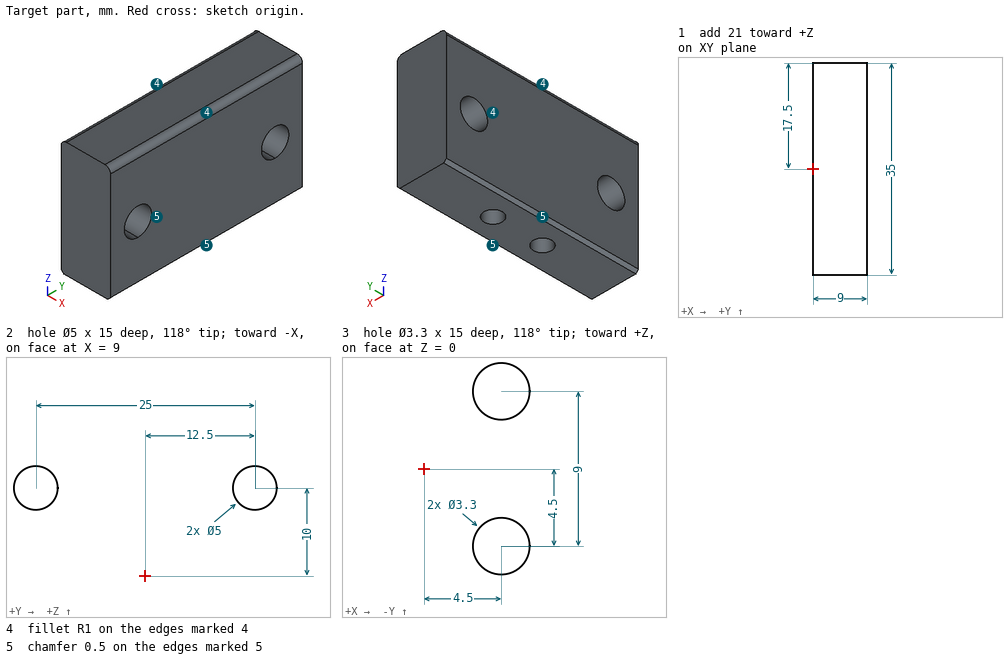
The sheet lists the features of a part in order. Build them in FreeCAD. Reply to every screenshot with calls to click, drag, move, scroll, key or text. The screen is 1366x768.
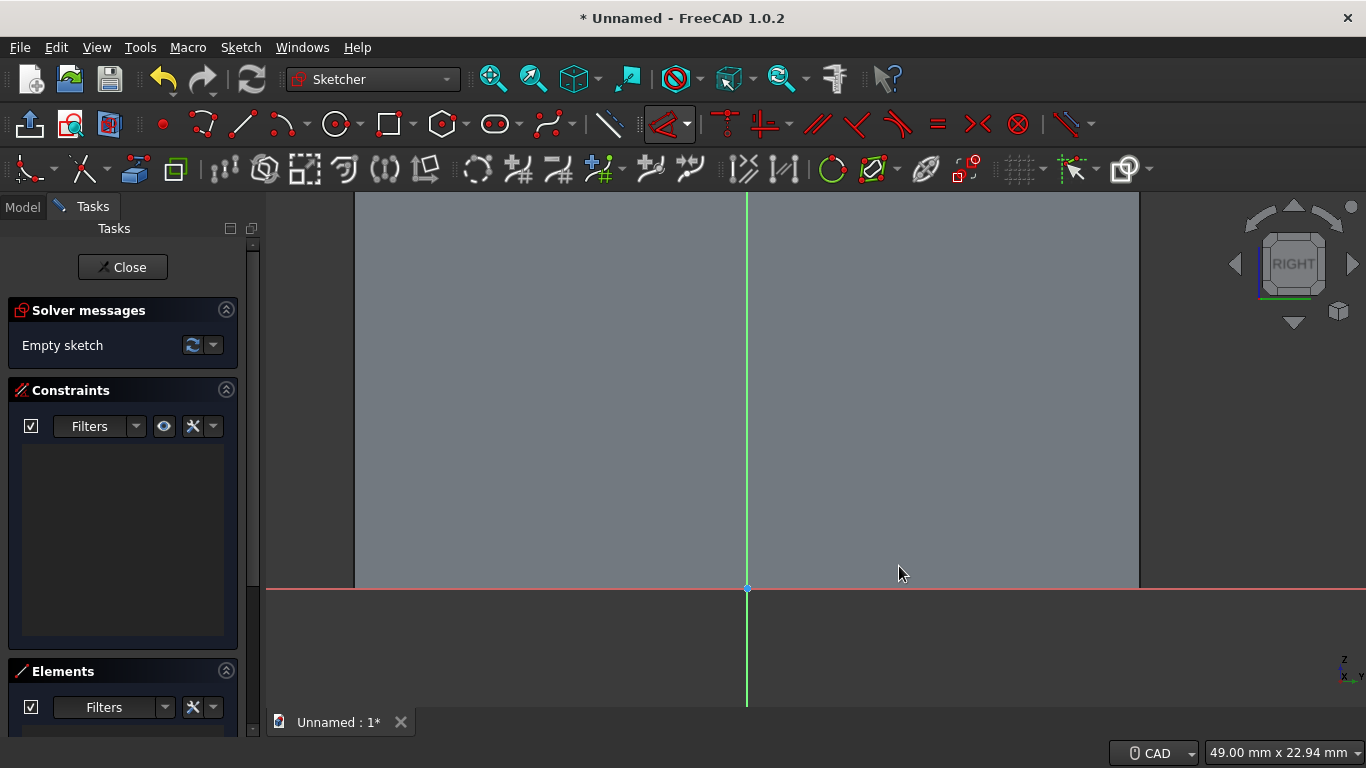
key(g)
key(c)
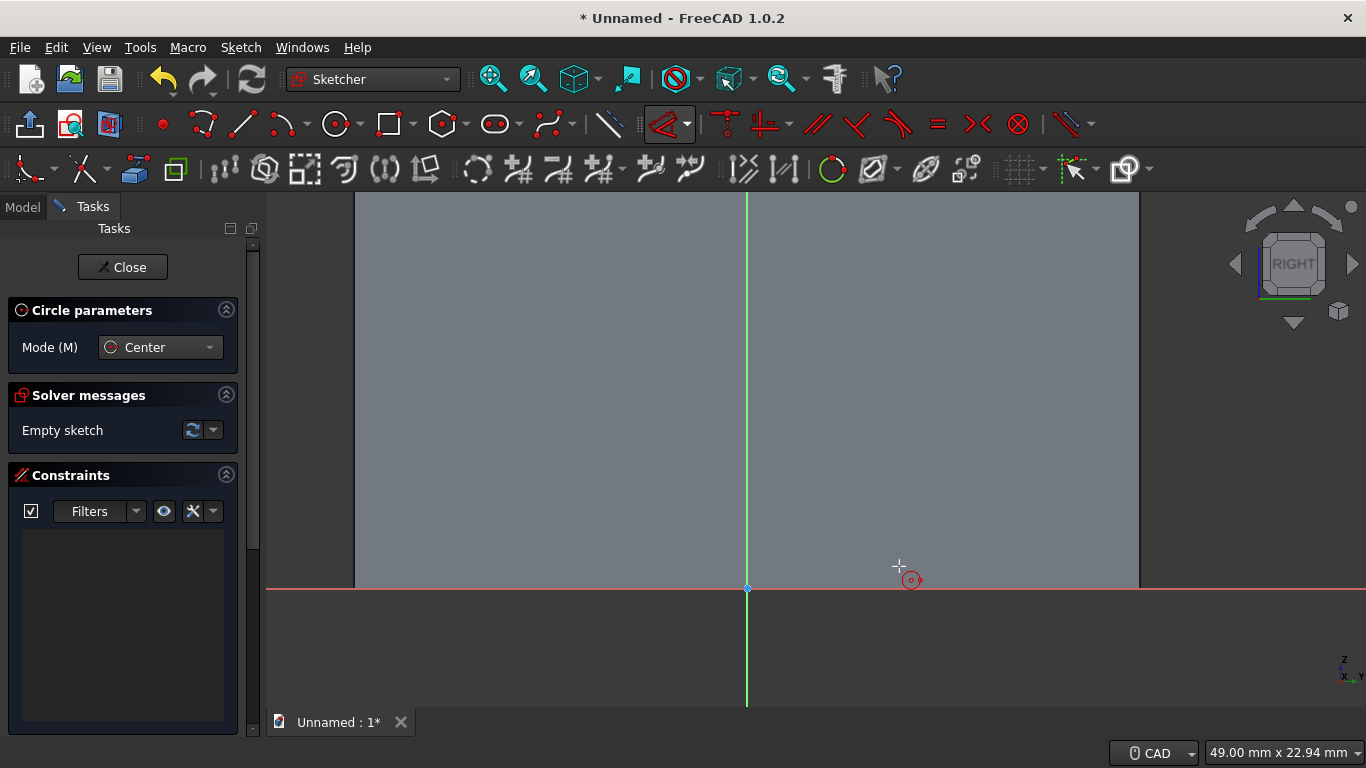
click(1028, 364)
move(1068, 325)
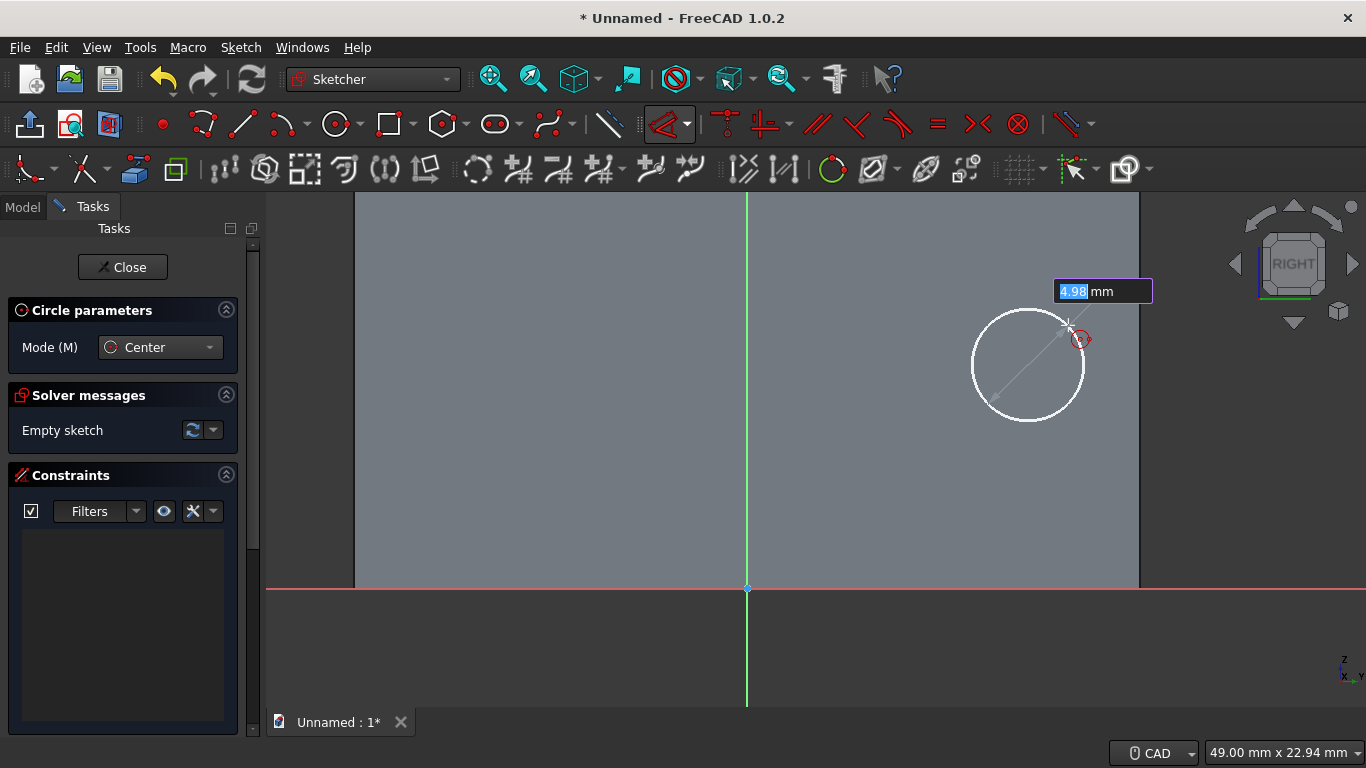
text(5)
key(Return)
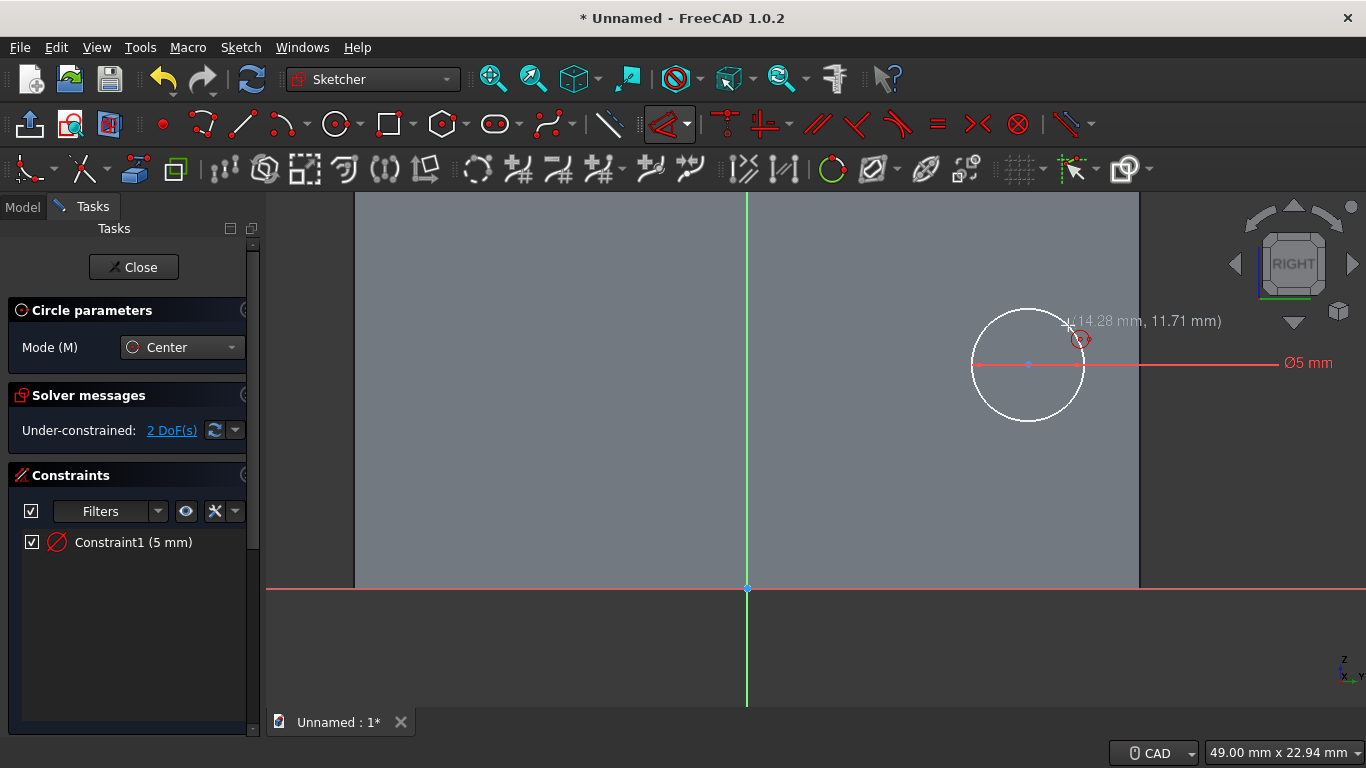
click(467, 364)
move(506, 325)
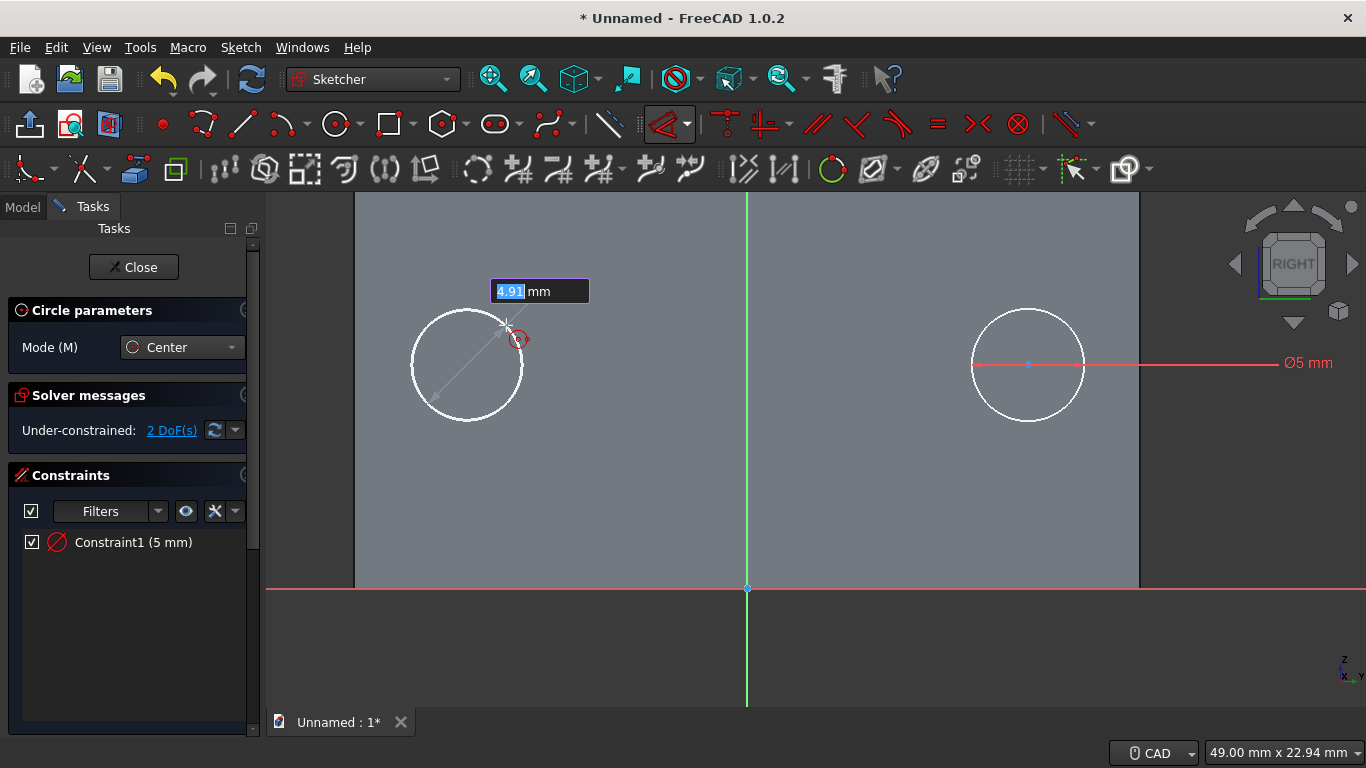
text(5)
key(Return)
key(Escape)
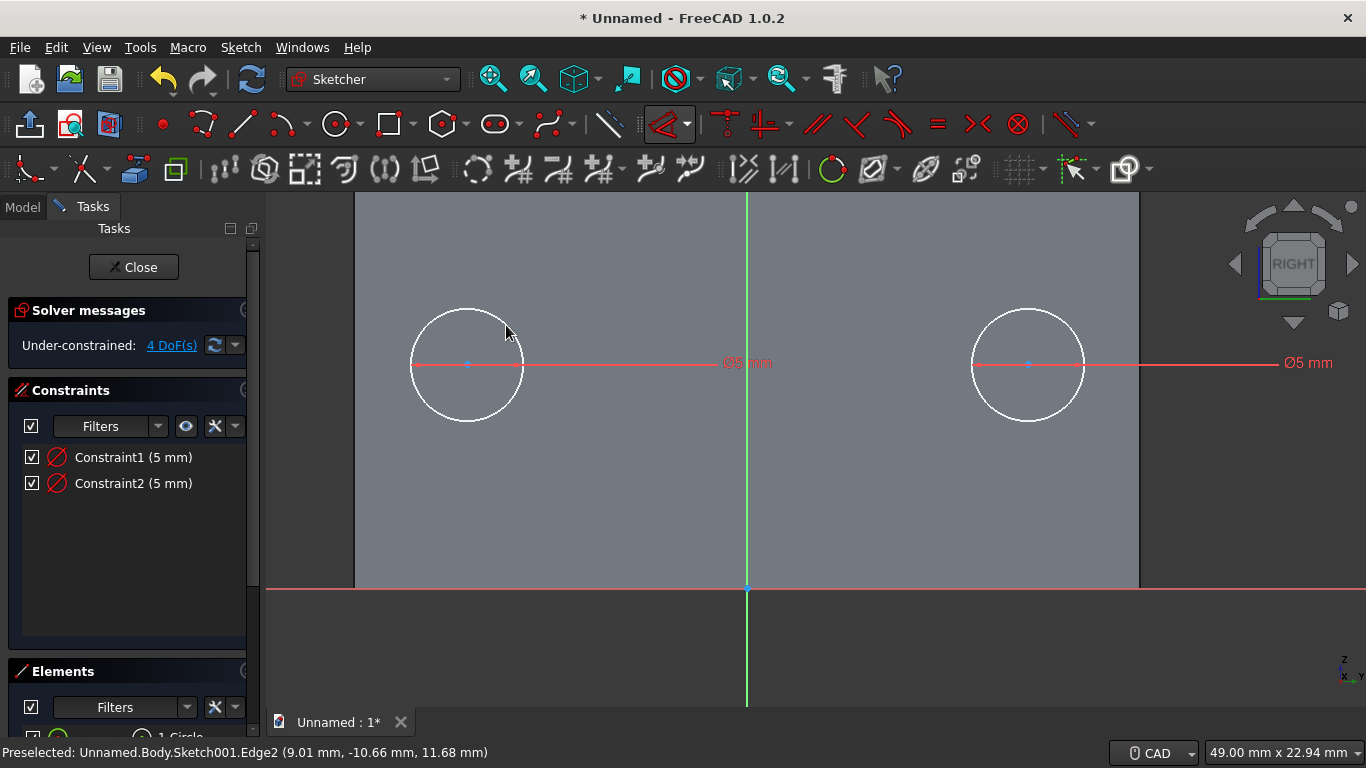
click(1028, 365)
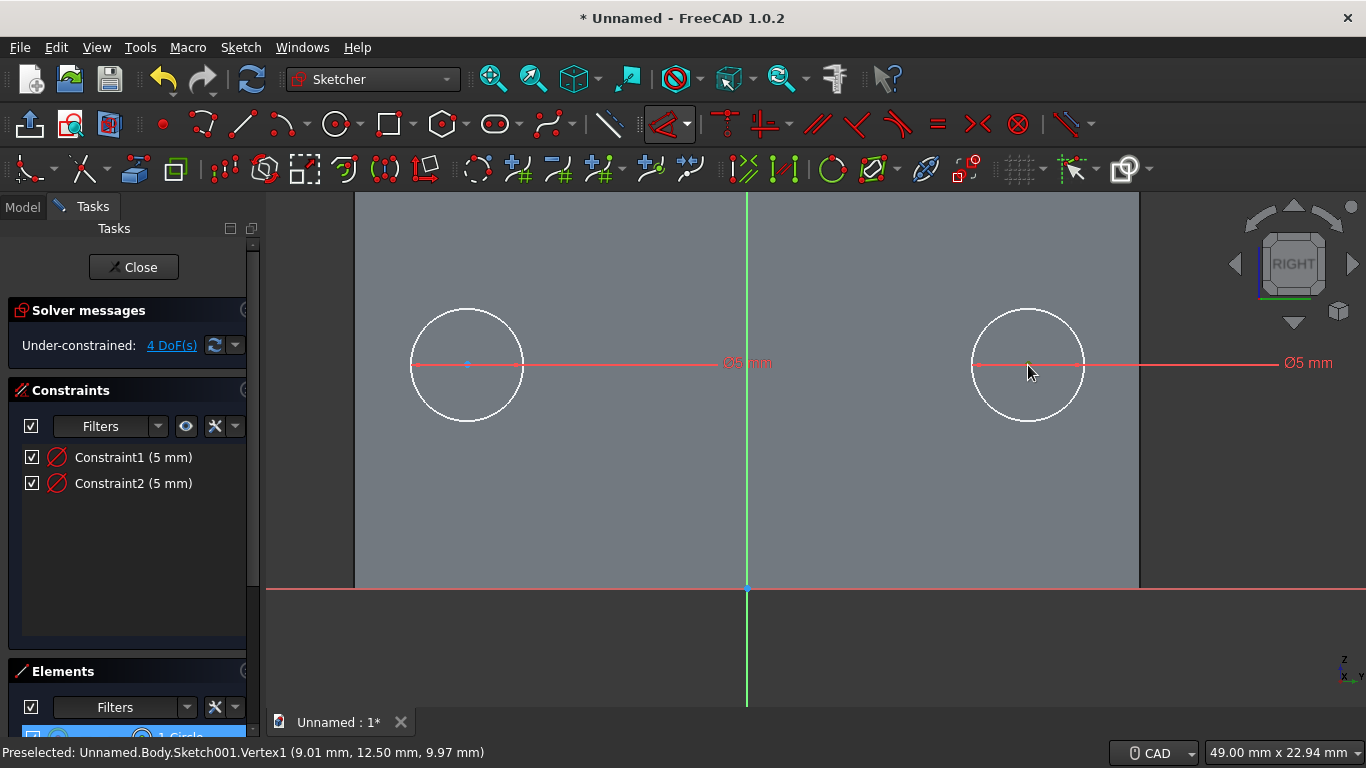
click(467, 365)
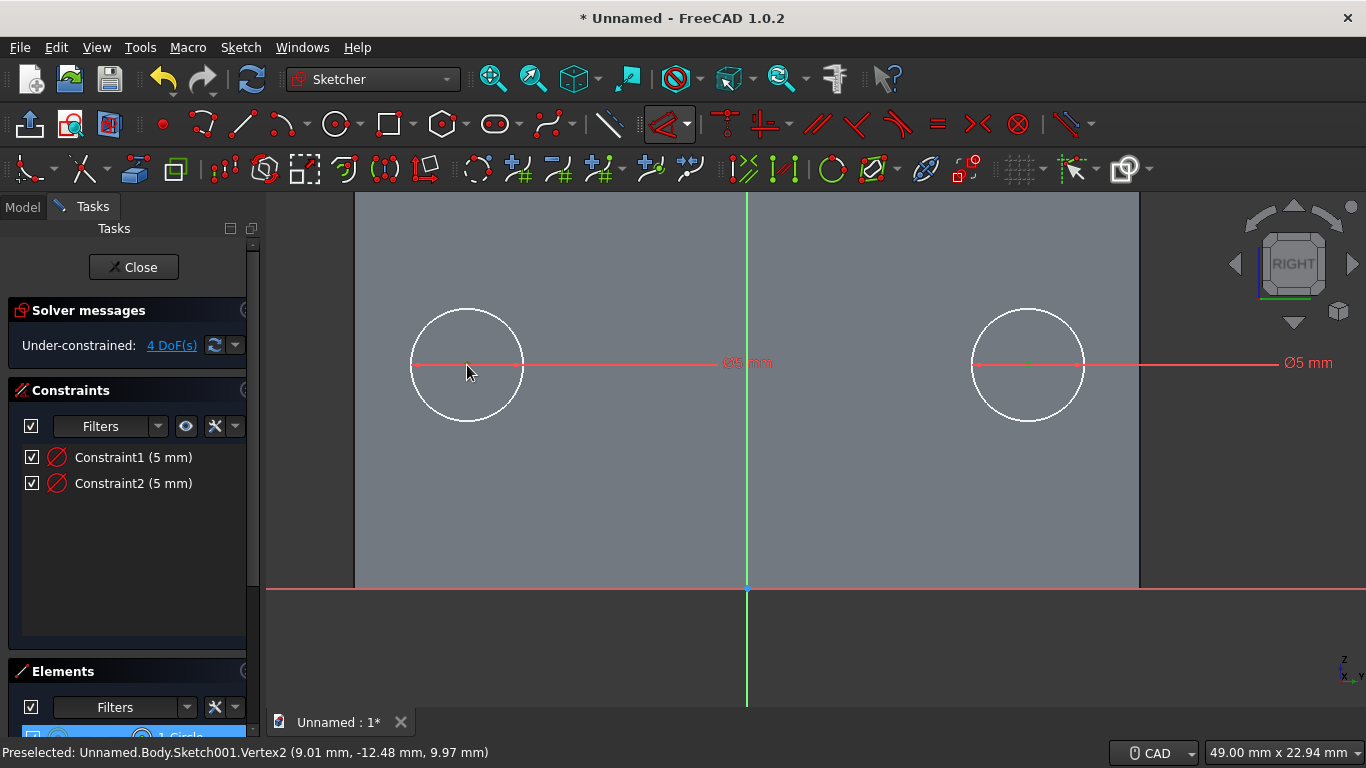
key(h)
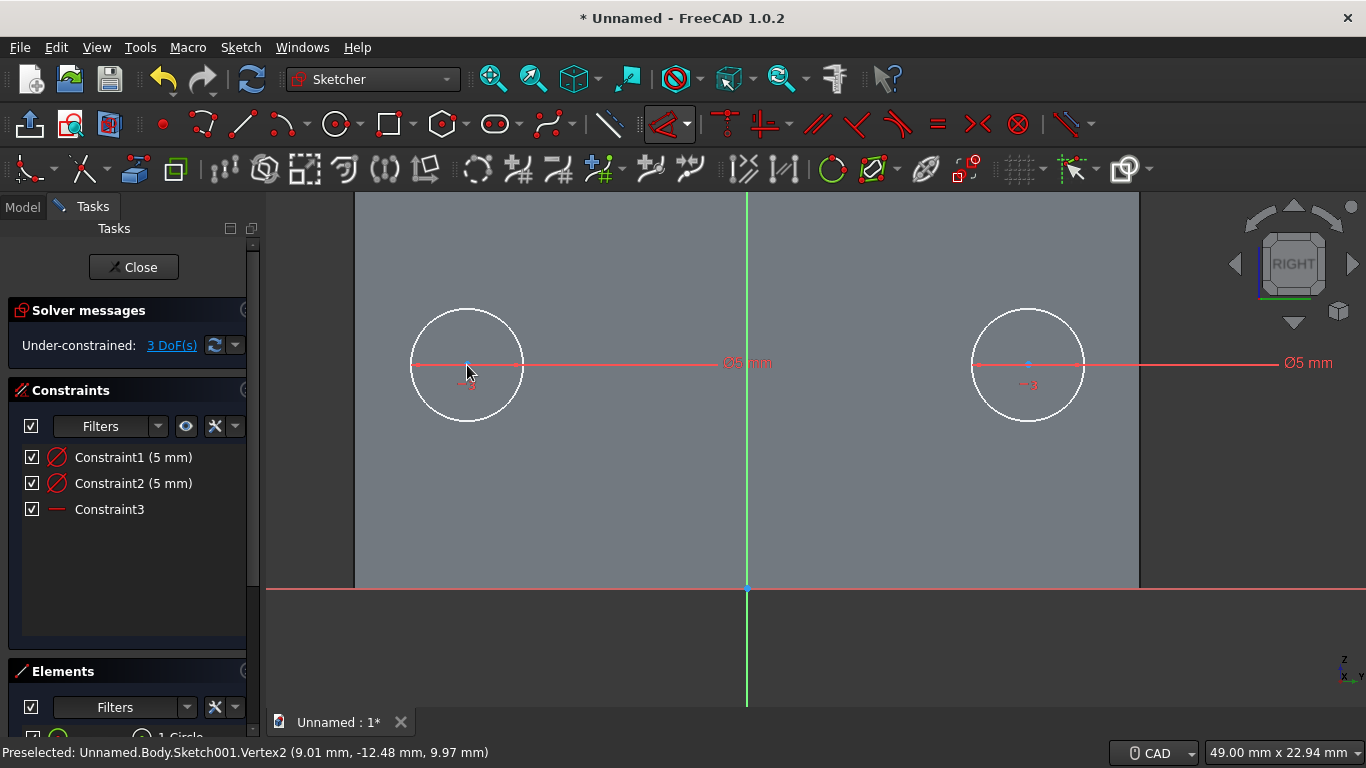
click(1028, 365)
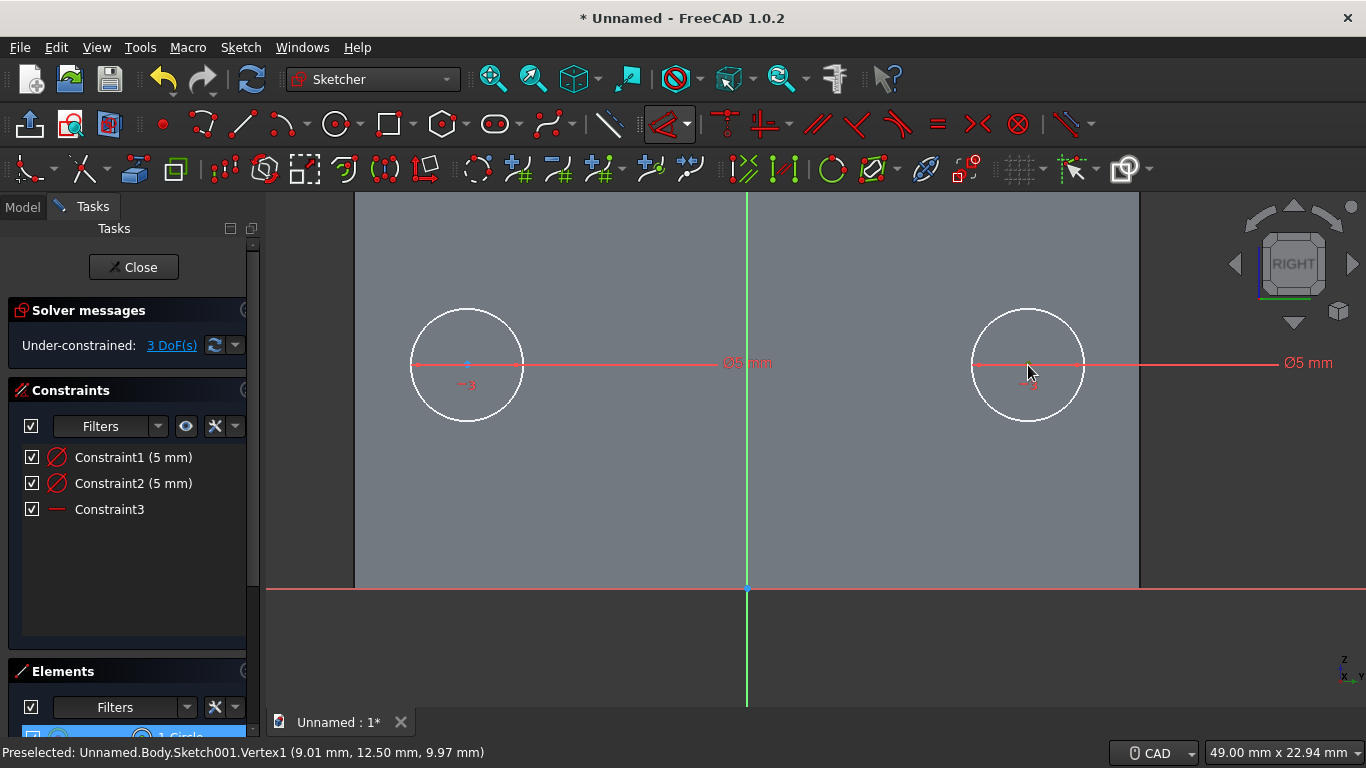
key(i)